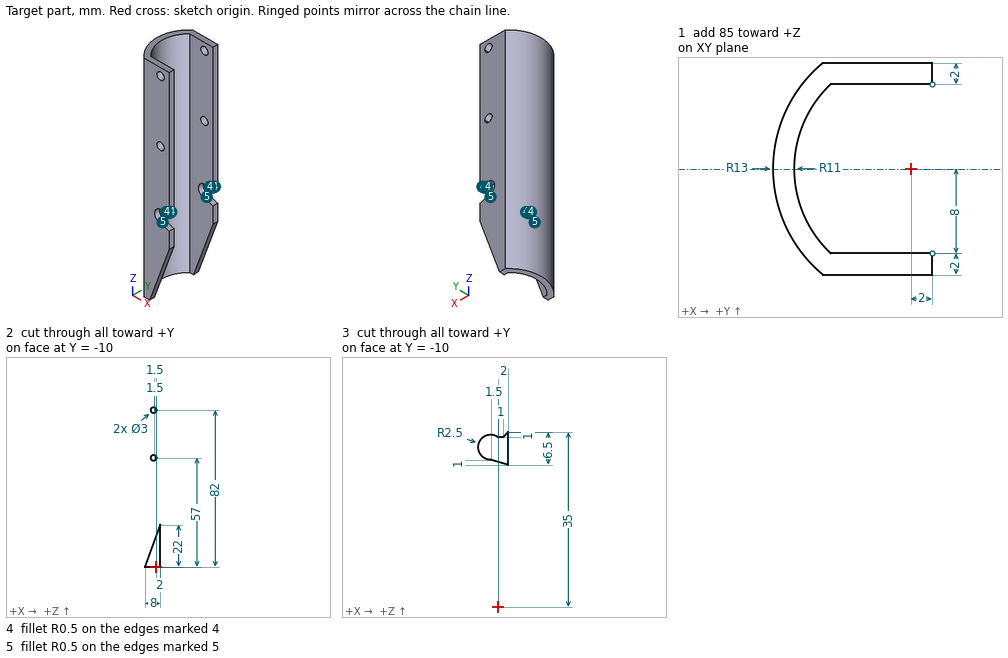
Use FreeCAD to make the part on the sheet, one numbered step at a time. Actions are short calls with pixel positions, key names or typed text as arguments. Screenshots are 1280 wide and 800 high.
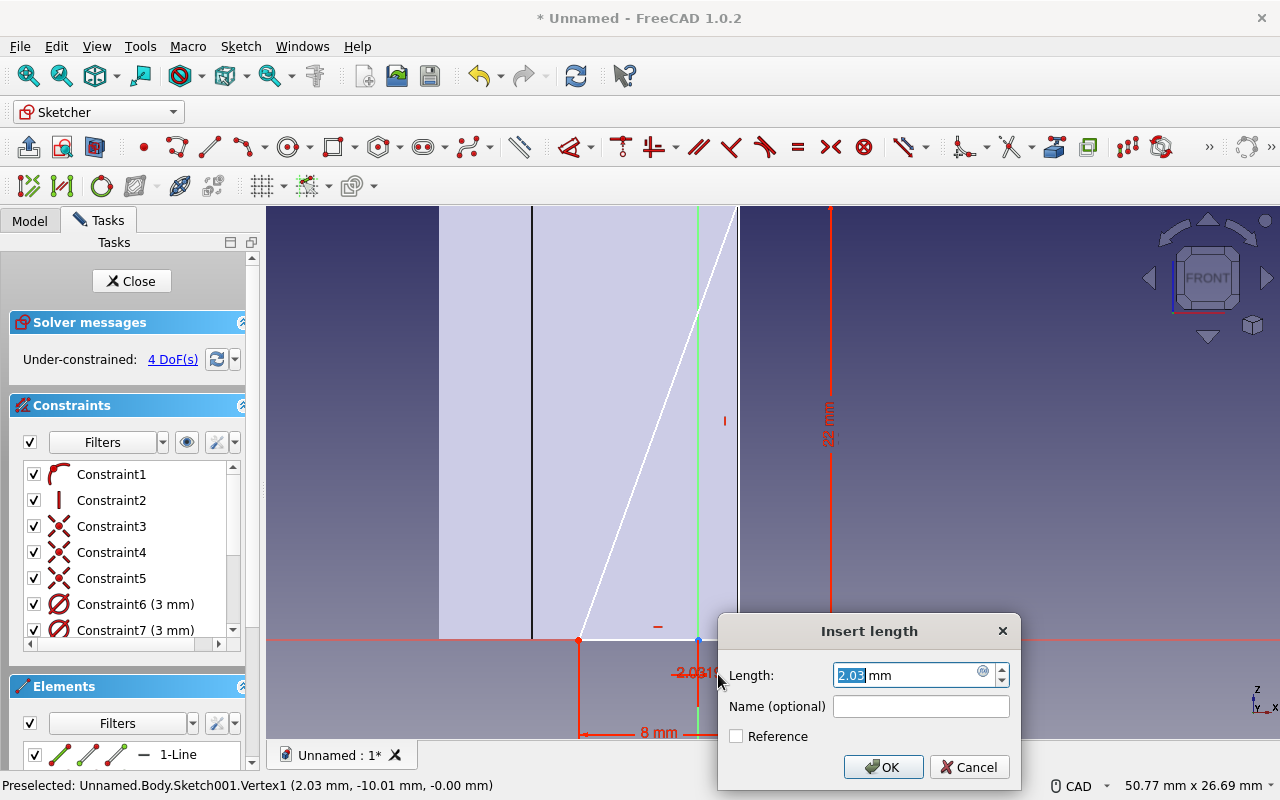
text(2)
key(Return)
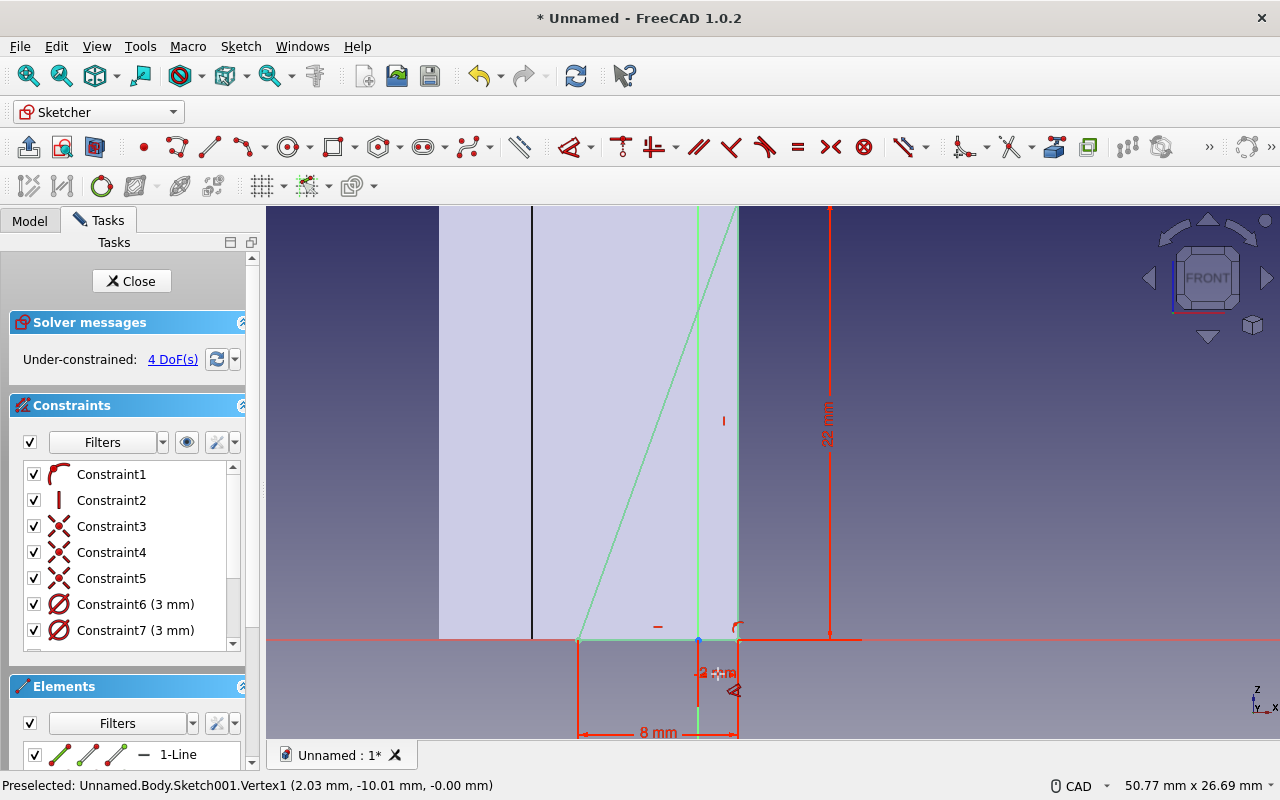
scroll(716, 641, down, 8)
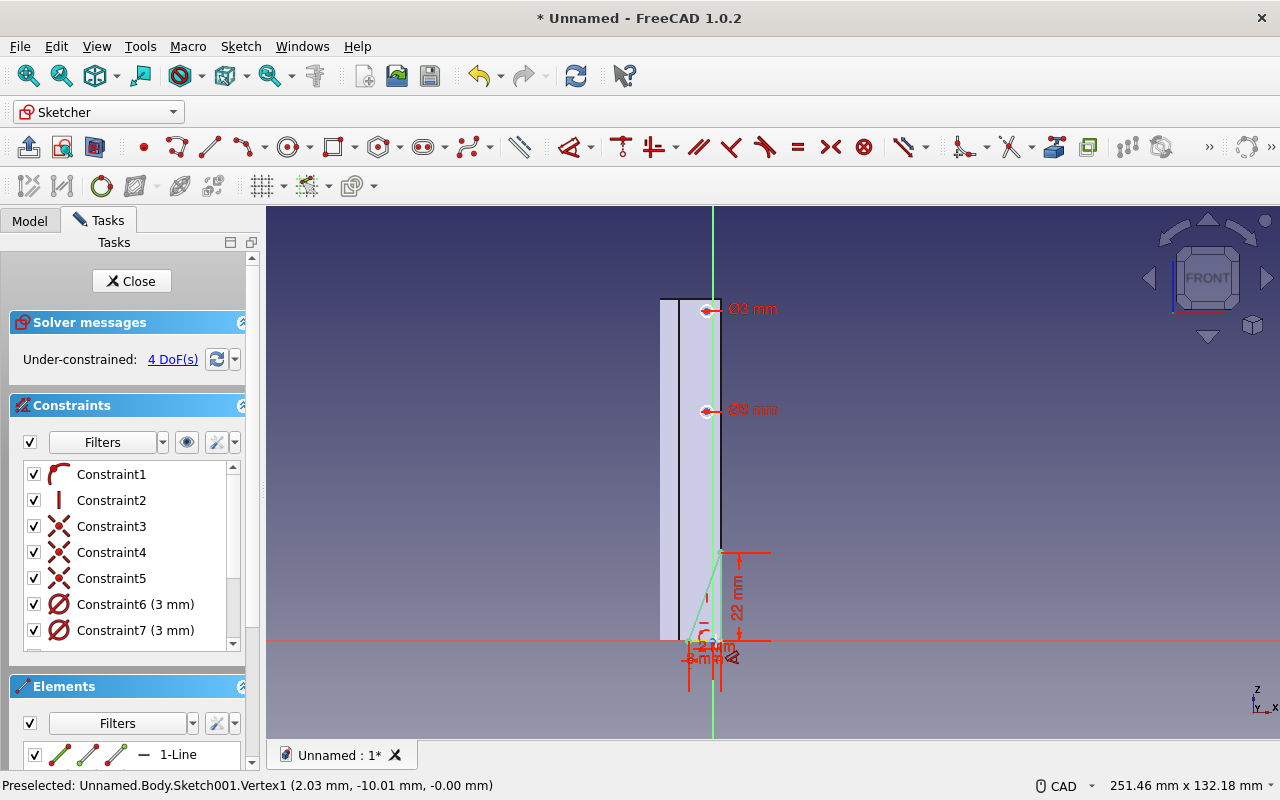
click(707, 311)
click(747, 476)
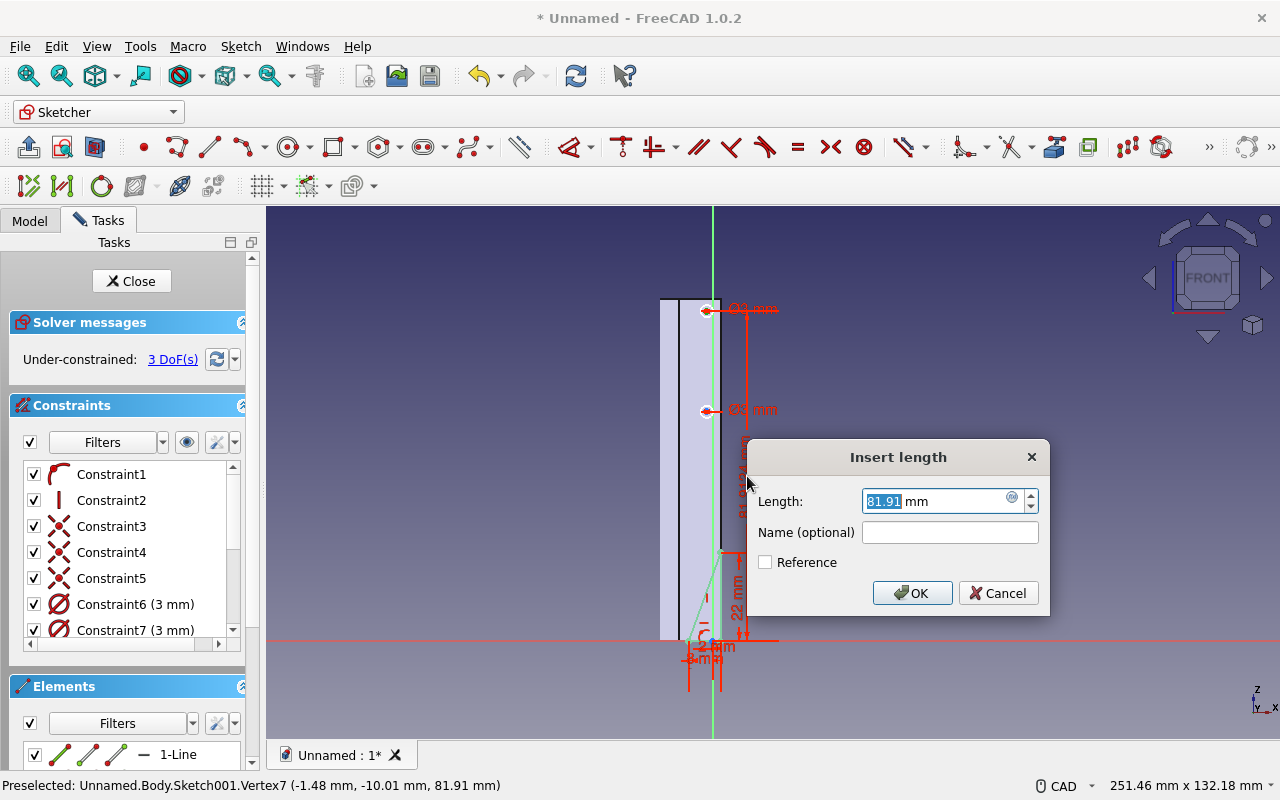
text(82)
key(Return)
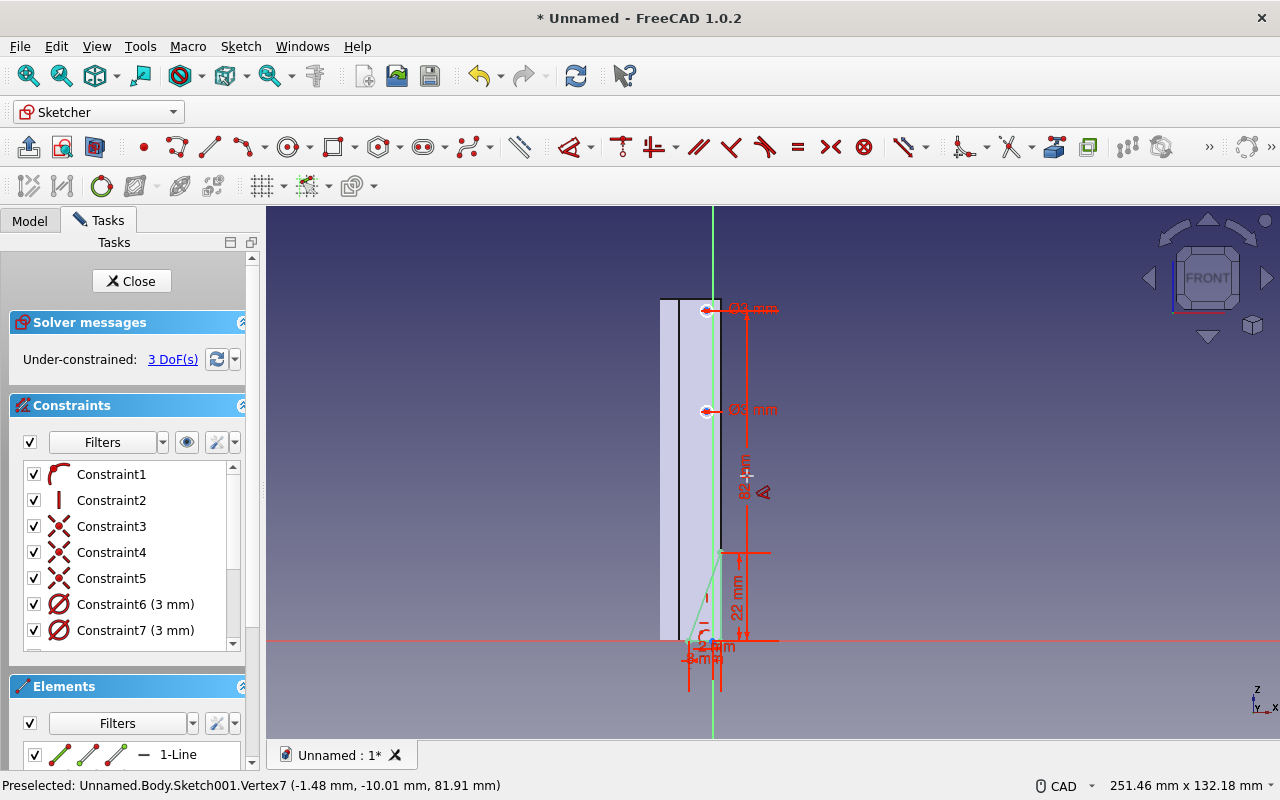
click(707, 412)
click(747, 527)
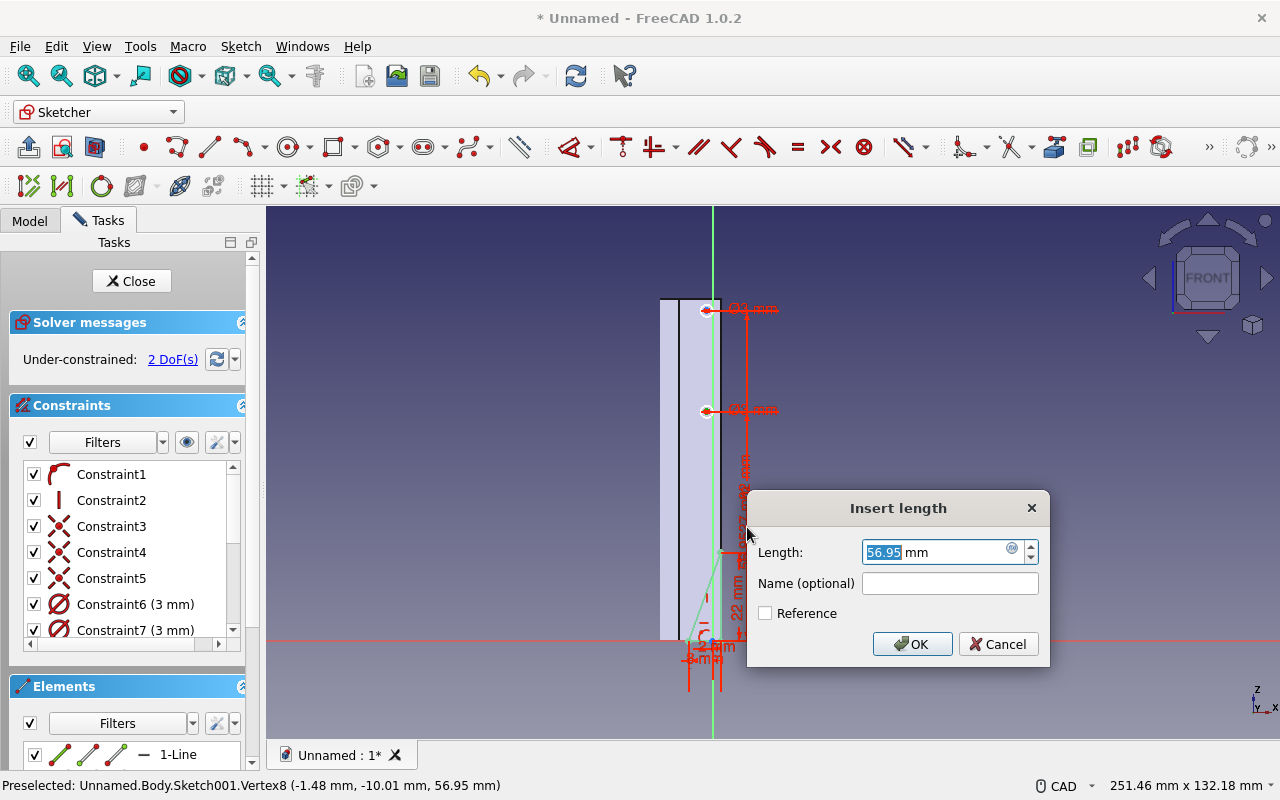
text(57)
key(Return)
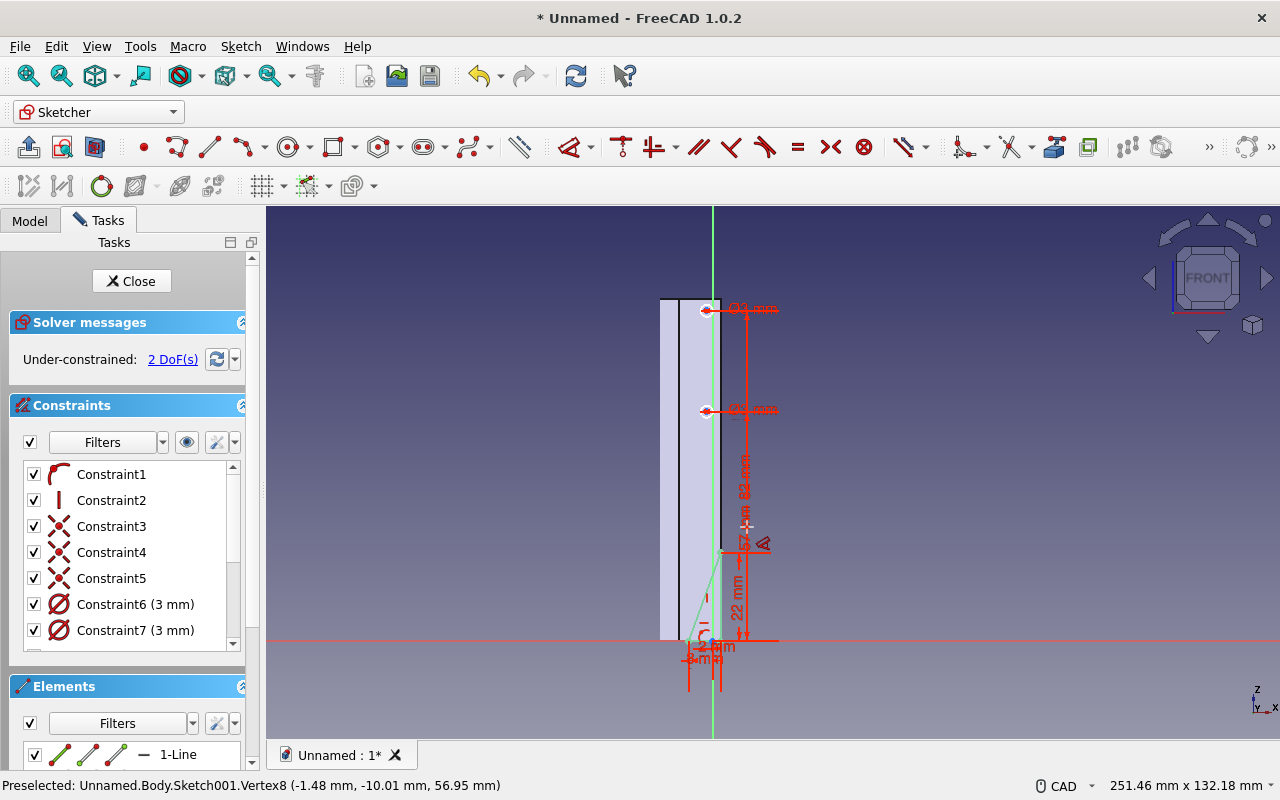
scroll(707, 311, up, 10)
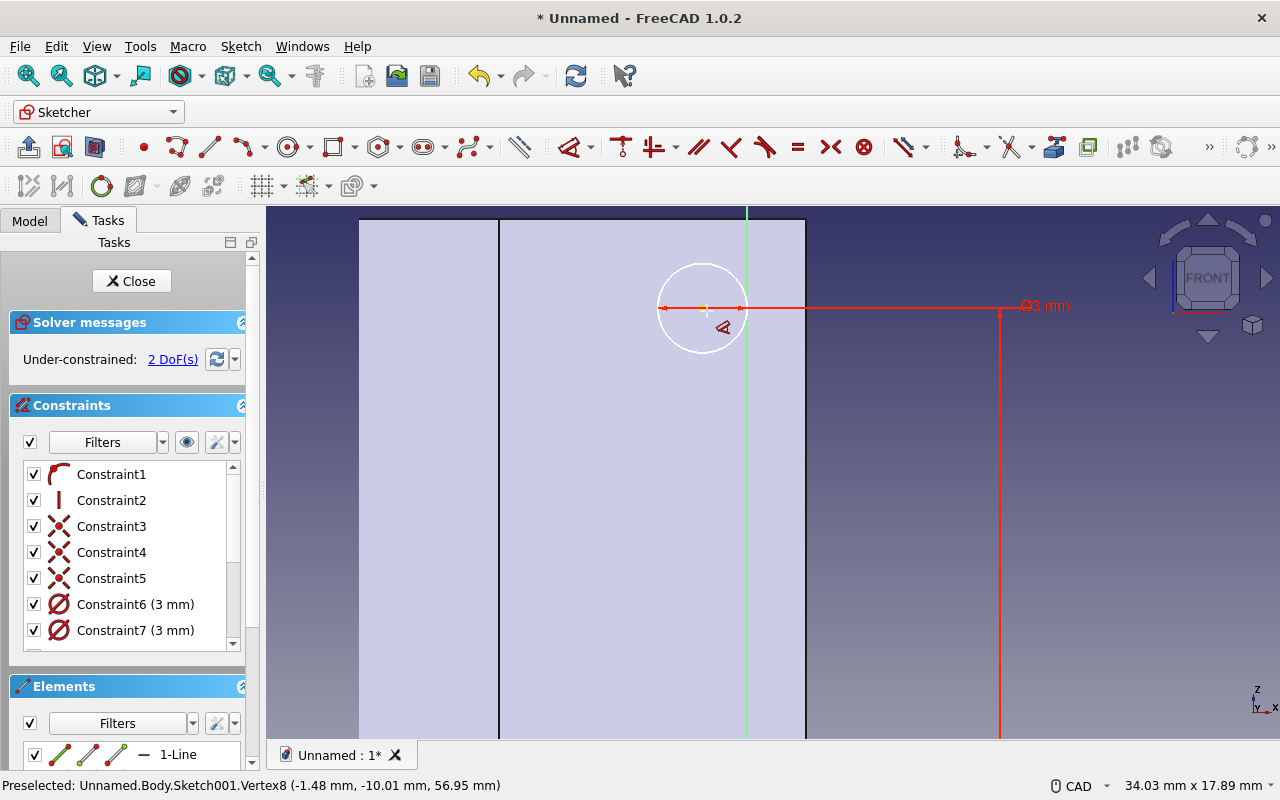
click(703, 308)
click(725, 250)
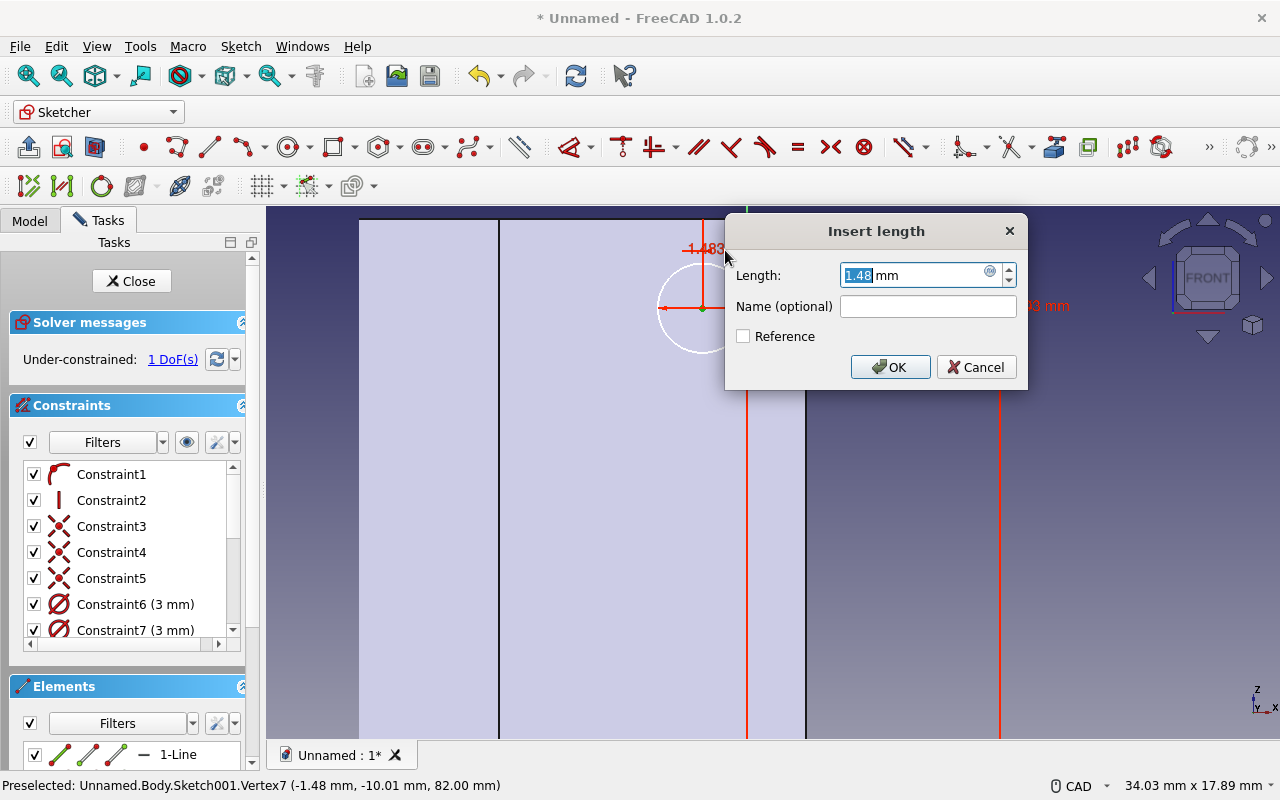
text(1.5)
key(Return)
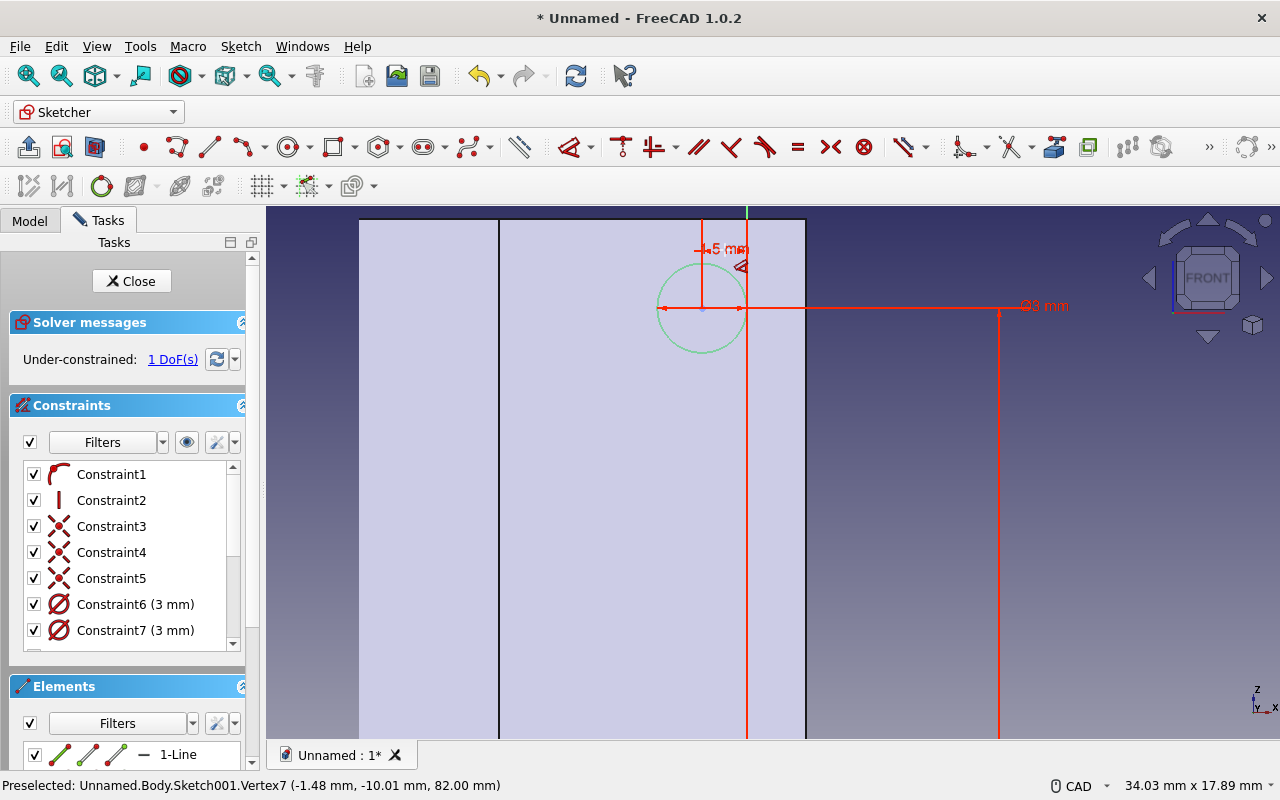
scroll(707, 310, down, 10)